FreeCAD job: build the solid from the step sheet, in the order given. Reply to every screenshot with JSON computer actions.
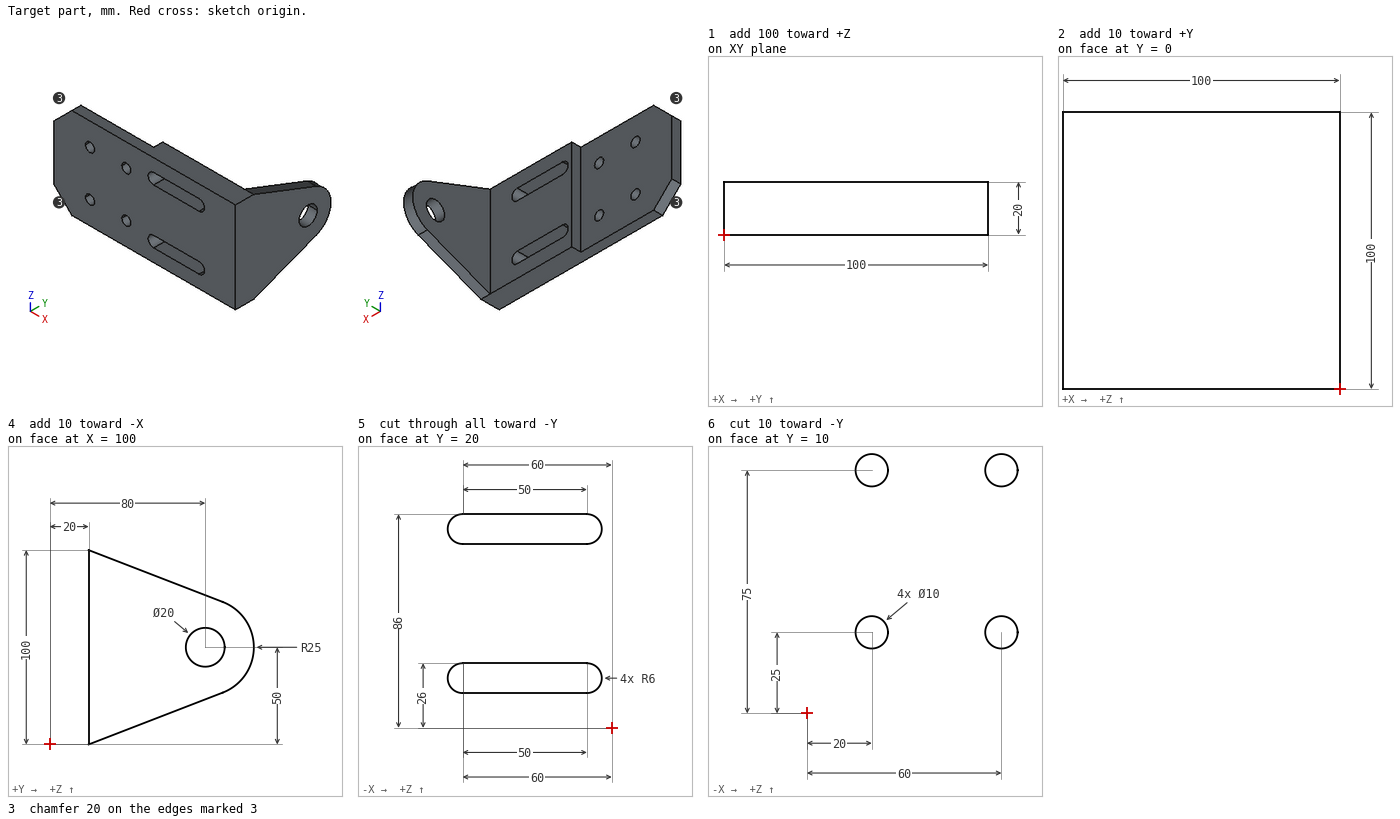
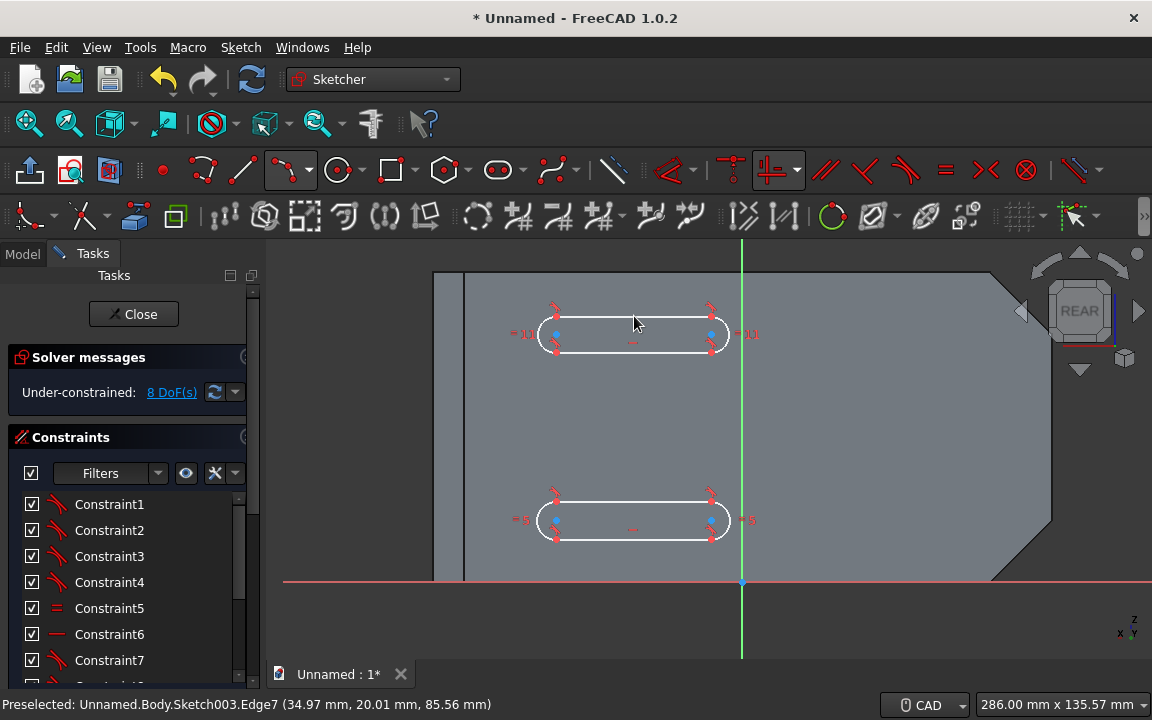
{"action": "left_click", "coordinate": [541, 510]}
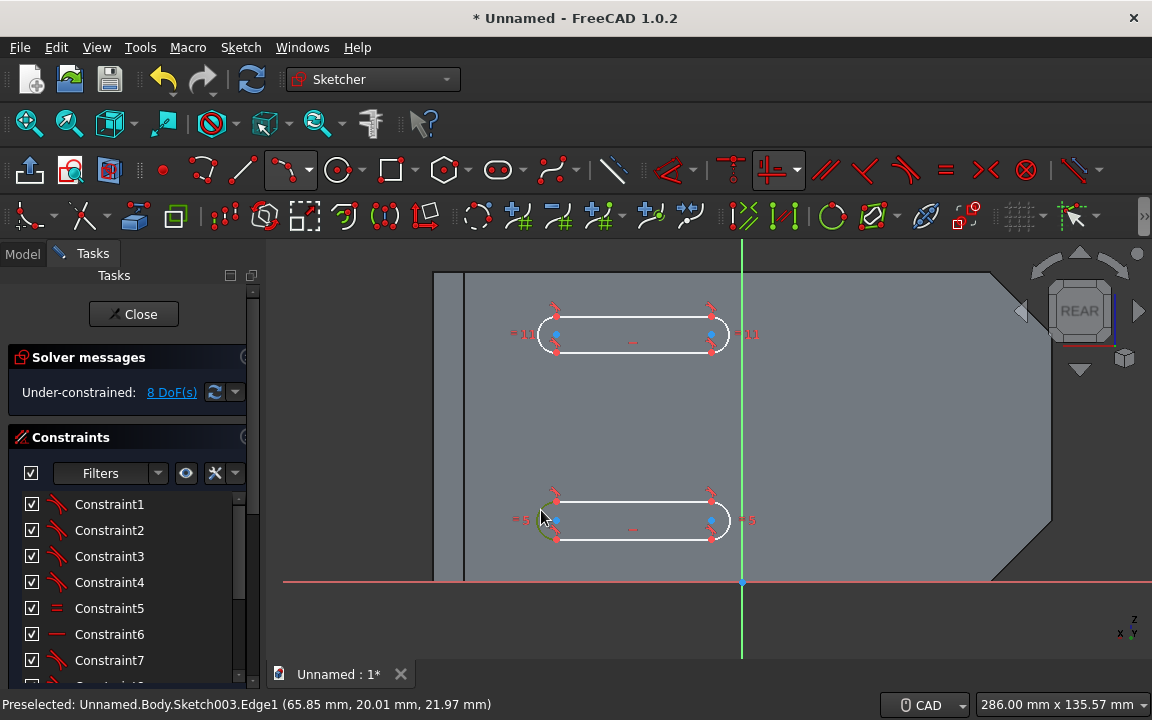
{"action": "left_click", "coordinate": [541, 324]}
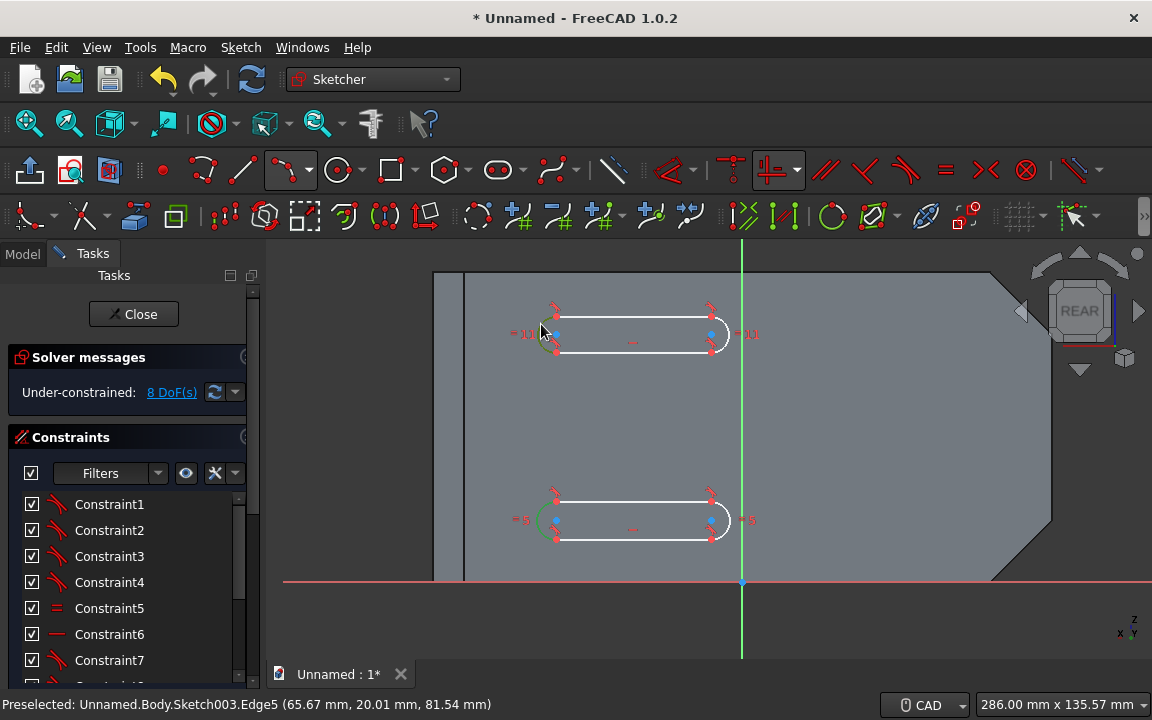
{"action": "left_click", "coordinate": [946, 170]}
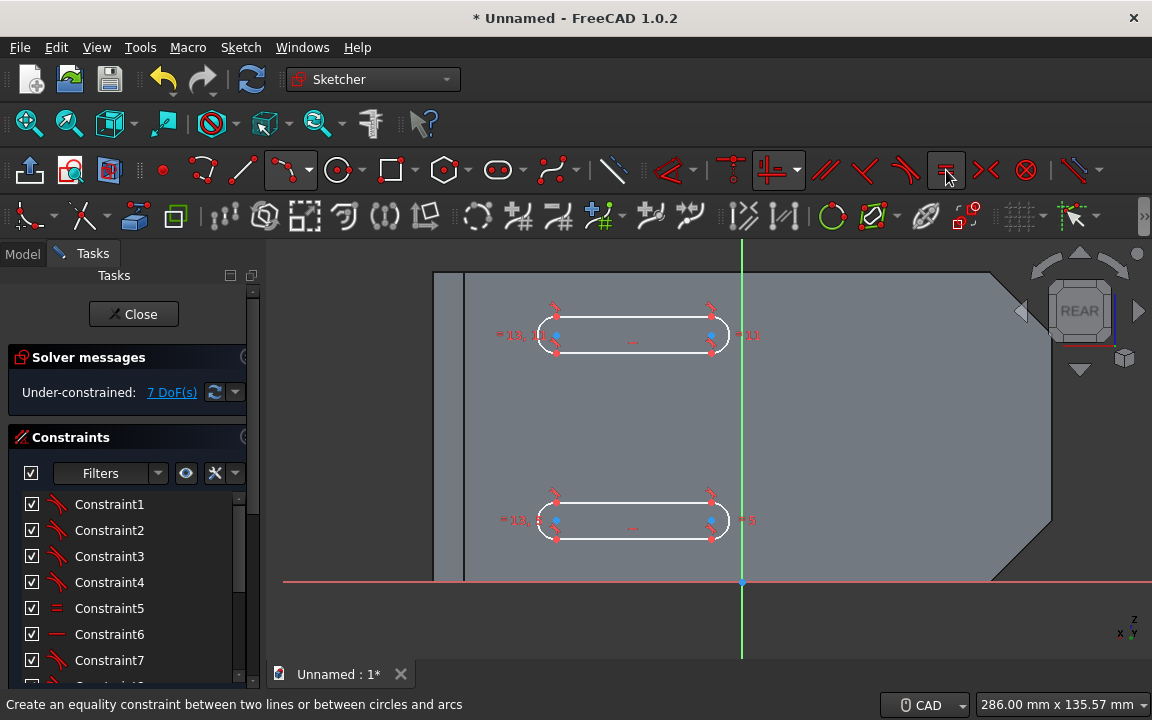
{"action": "left_click", "coordinate": [668, 170]}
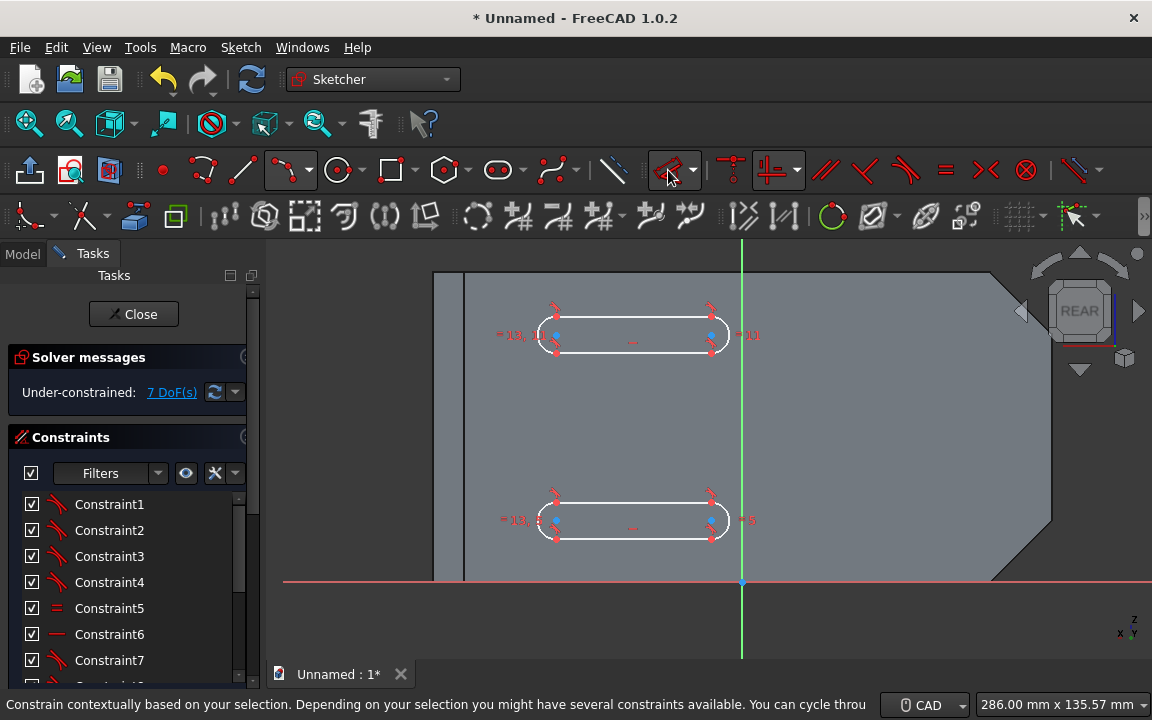
{"action": "scroll", "coordinate": [541, 510], "scroll_direction": "up", "scroll_amount": 4}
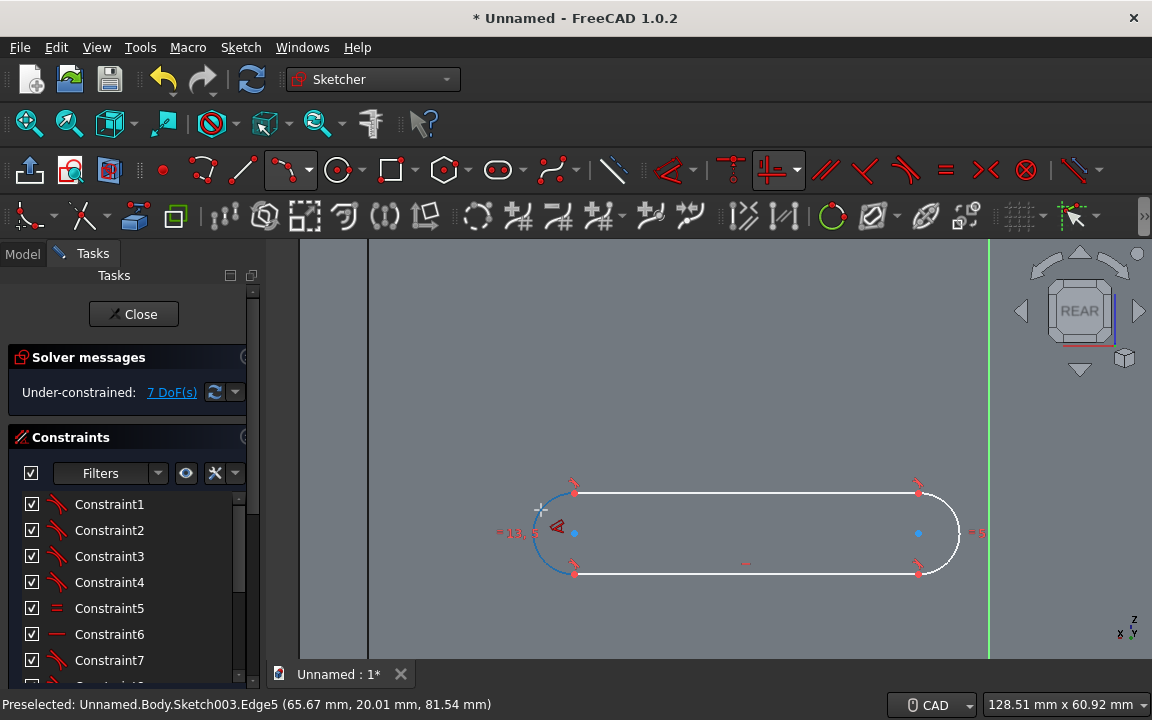
{"action": "left_click", "coordinate": [541, 510]}
{"action": "left_click", "coordinate": [515, 491]}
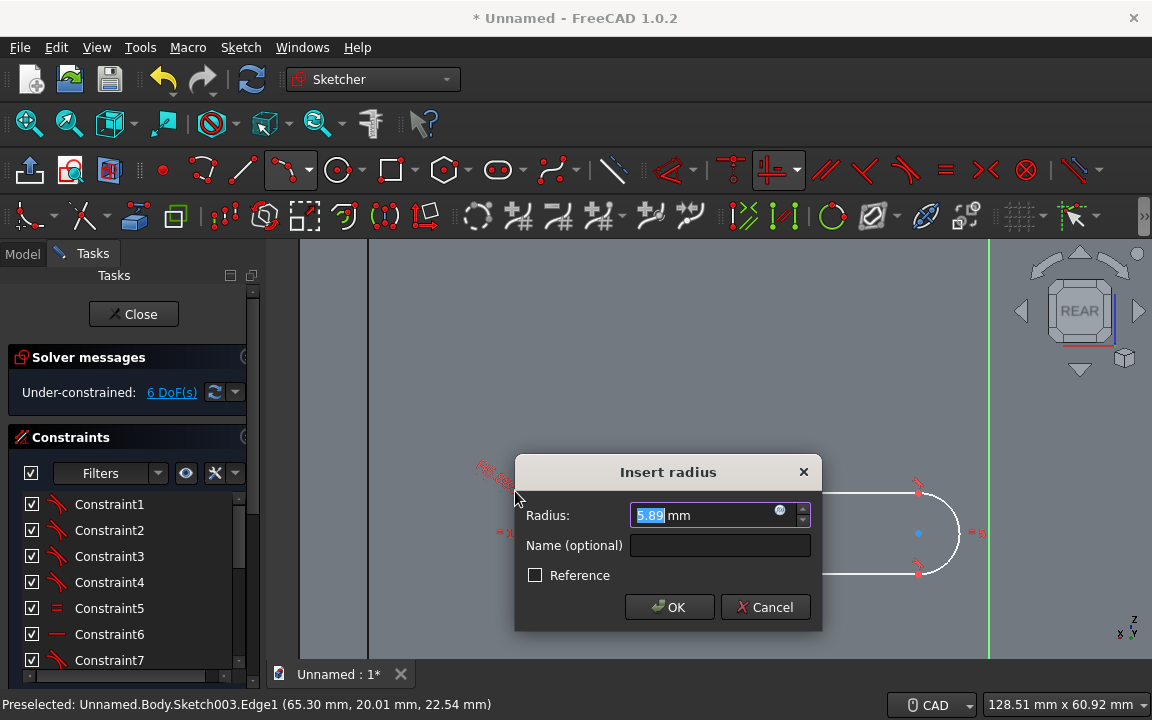
{"action": "type", "text": "6"}
{"action": "key", "text": "Return"}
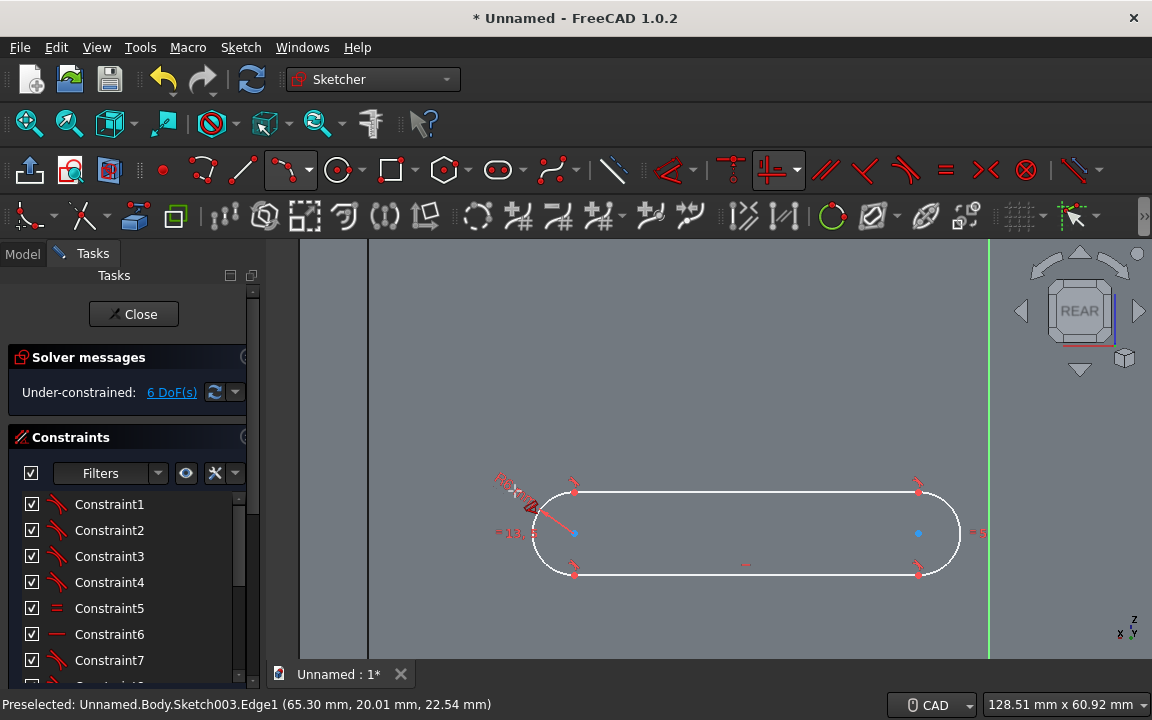
{"action": "left_click", "coordinate": [677, 492]}
{"action": "left_click", "coordinate": [746, 526]}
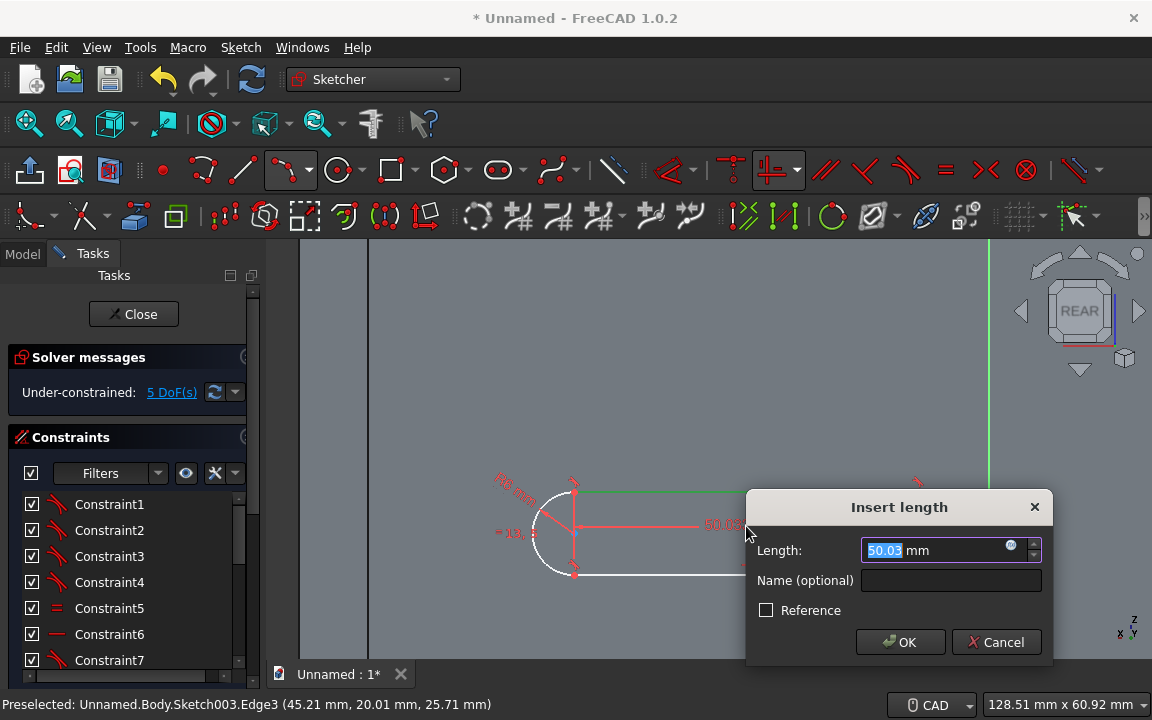
{"action": "type", "text": "50"}
{"action": "key", "text": "Return"}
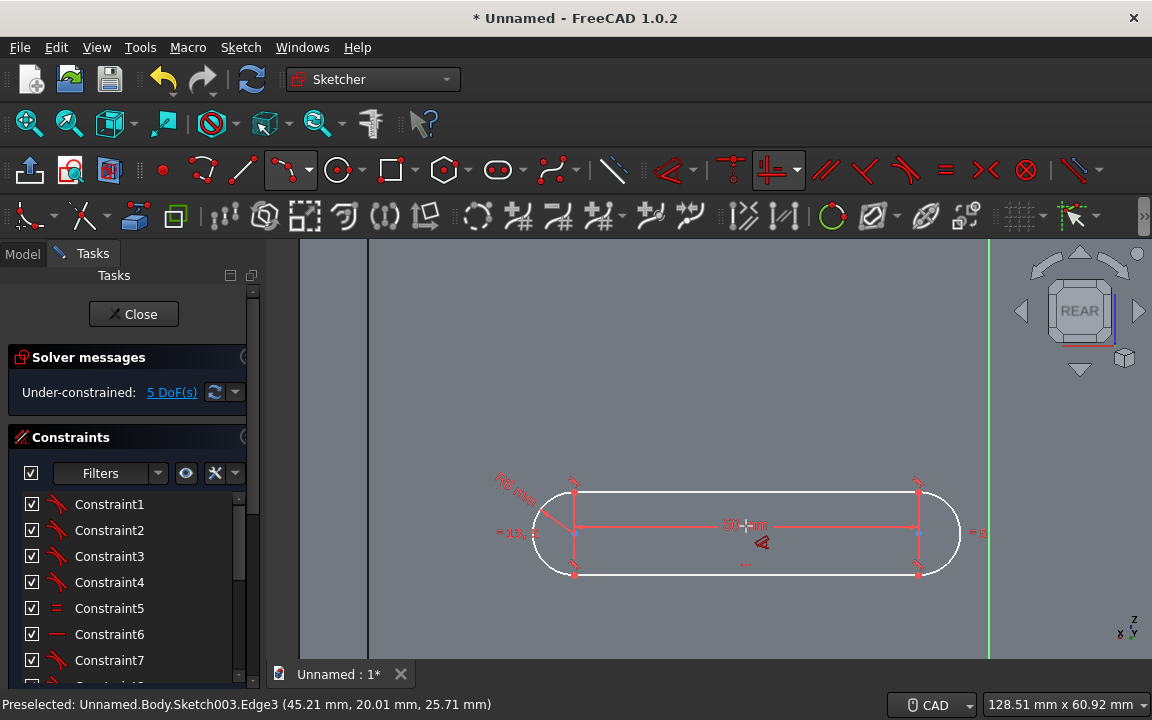
{"action": "scroll", "coordinate": [542, 511], "scroll_direction": "down", "scroll_amount": 4}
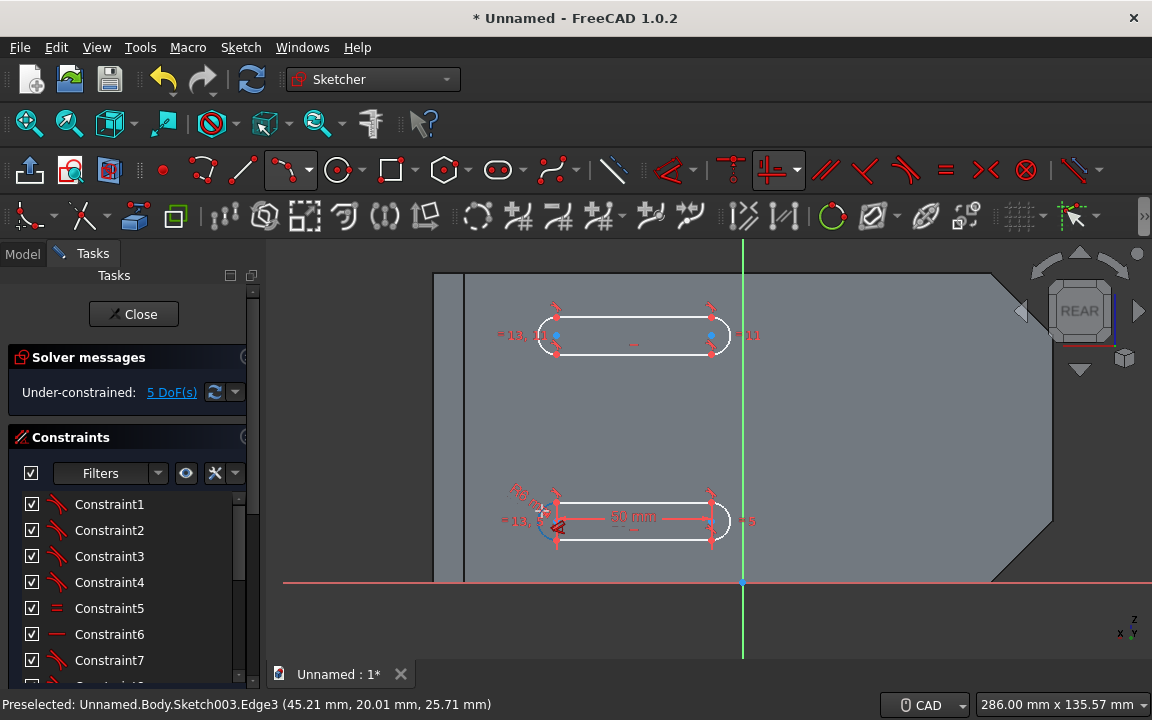
{"action": "left_click", "coordinate": [603, 317]}
{"action": "left_click", "coordinate": [634, 283]}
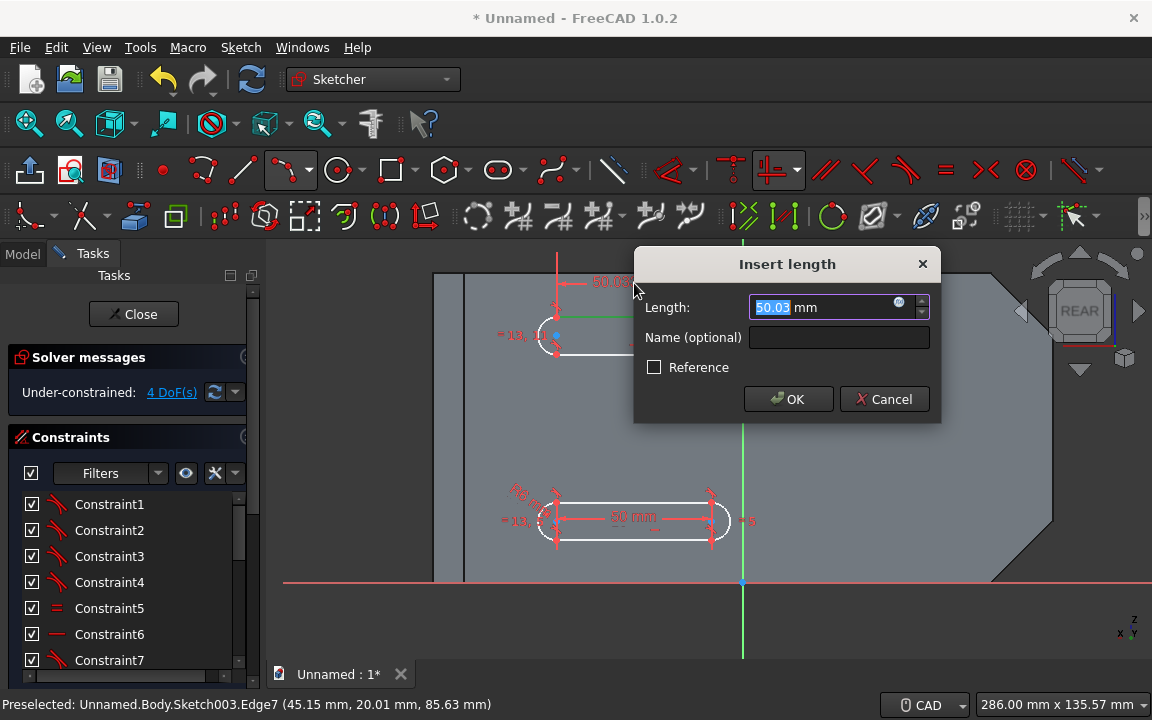
{"action": "type", "text": "50"}
{"action": "key", "text": "Return"}